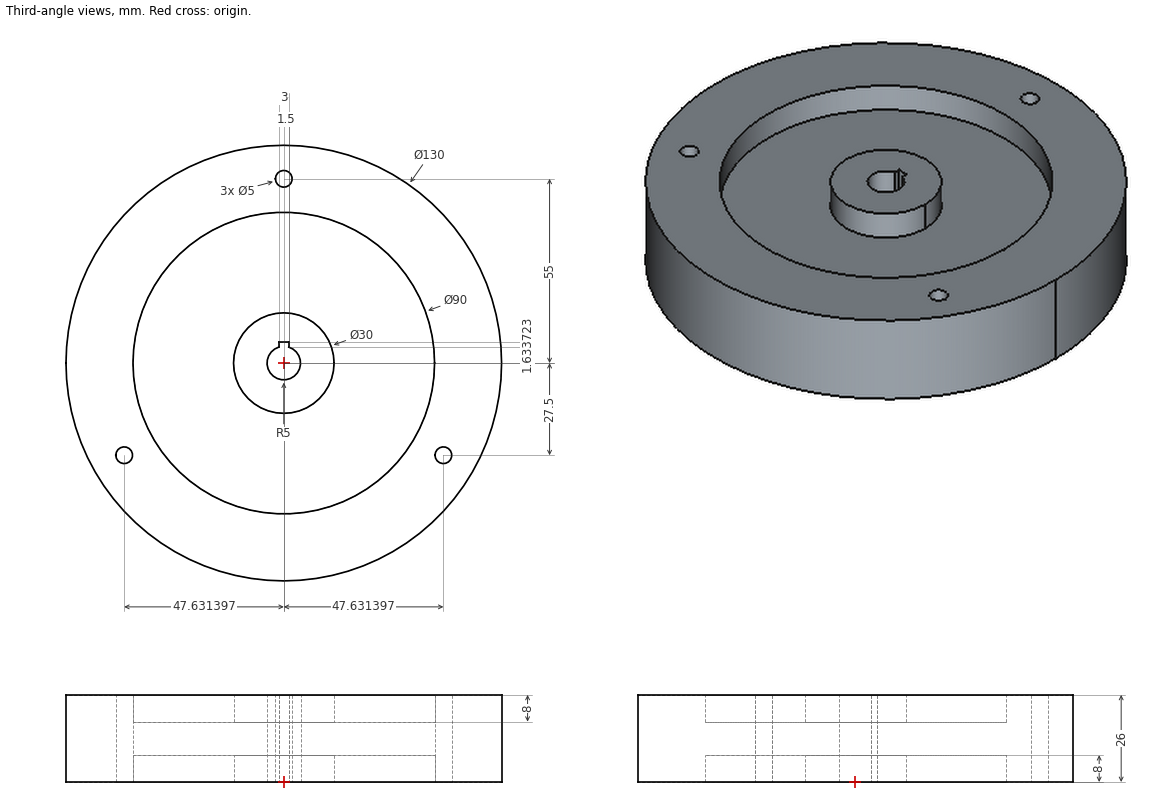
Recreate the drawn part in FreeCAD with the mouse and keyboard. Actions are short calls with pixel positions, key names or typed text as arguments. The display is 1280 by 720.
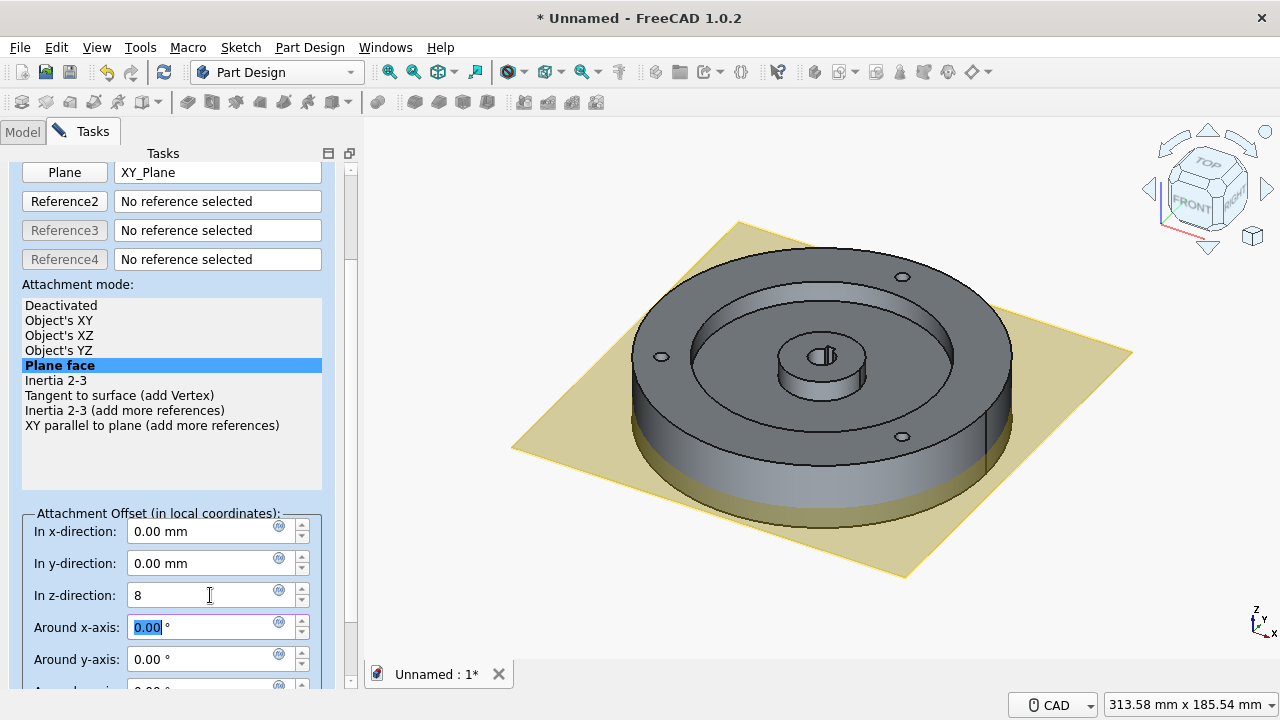
scroll(351, 426, up, 3)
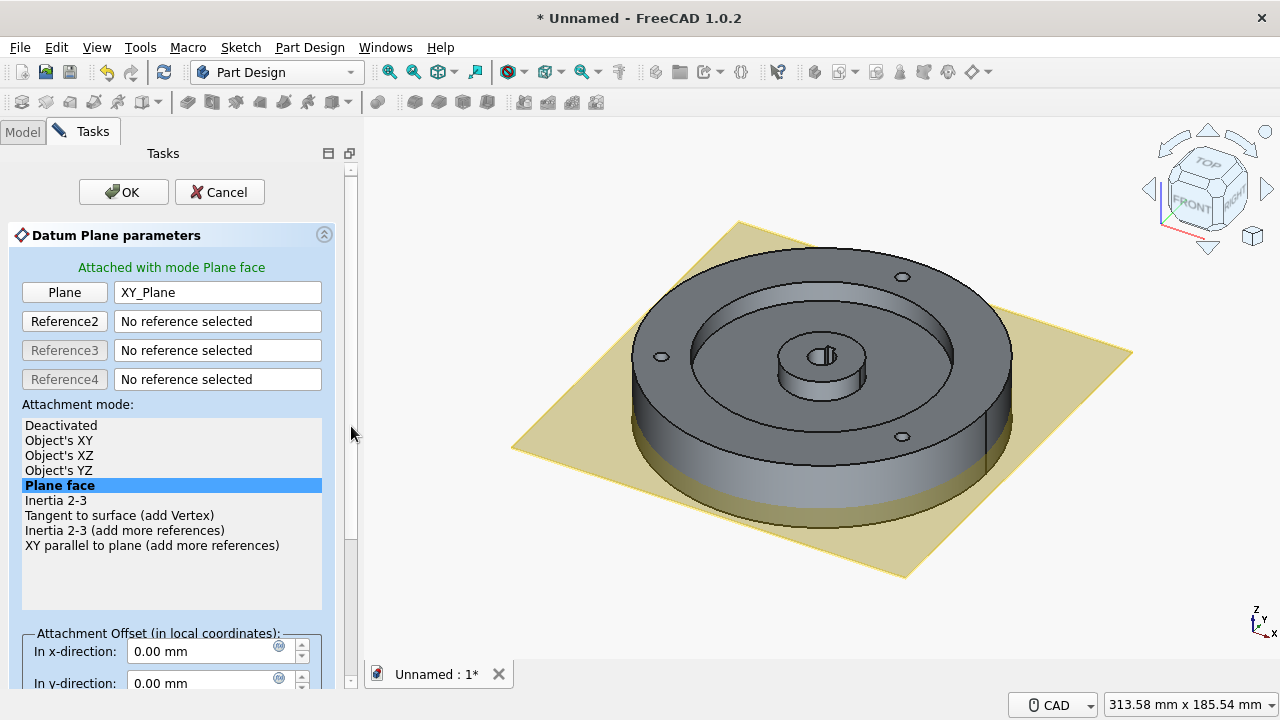
click(124, 192)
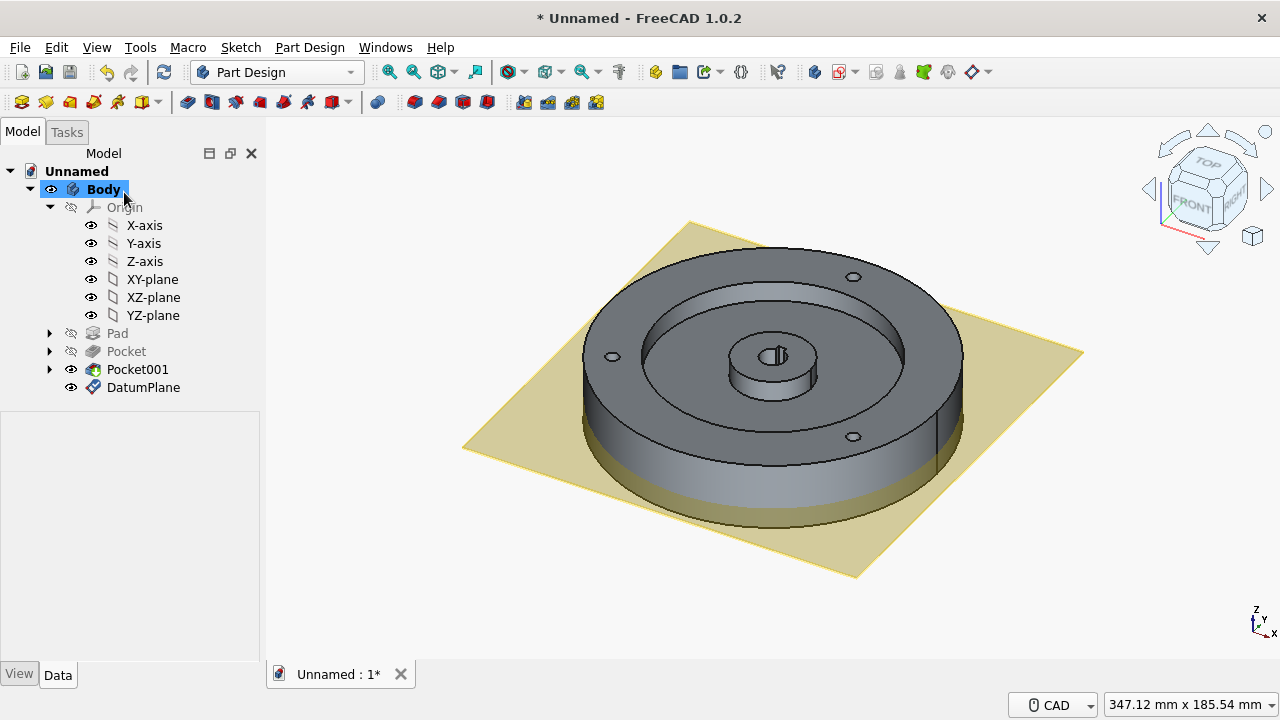
click(116, 387)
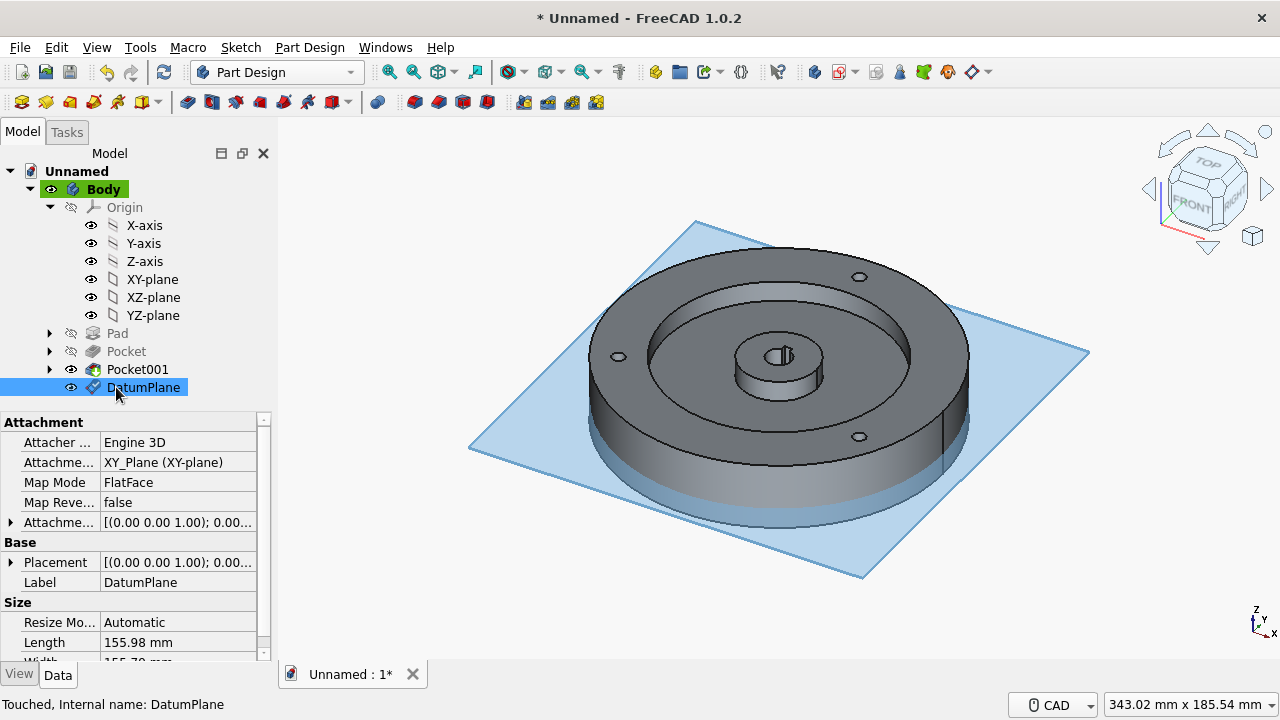
click(840, 72)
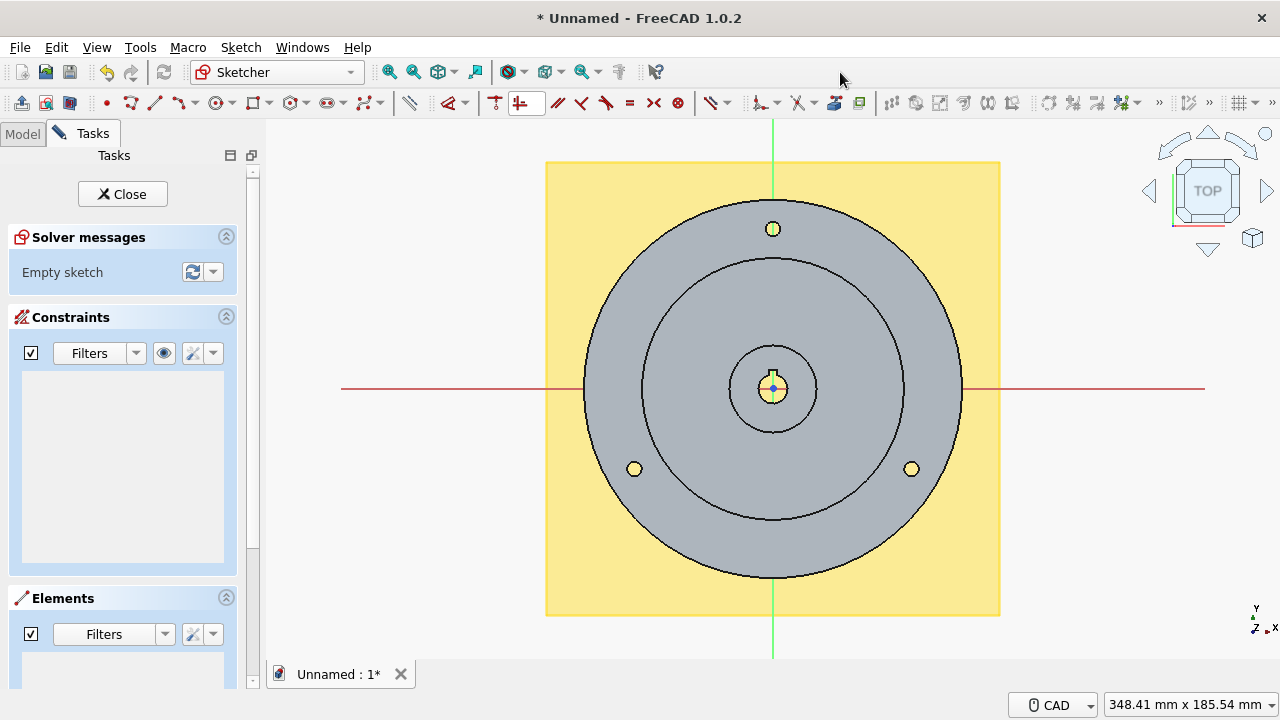
key(q)
key(s)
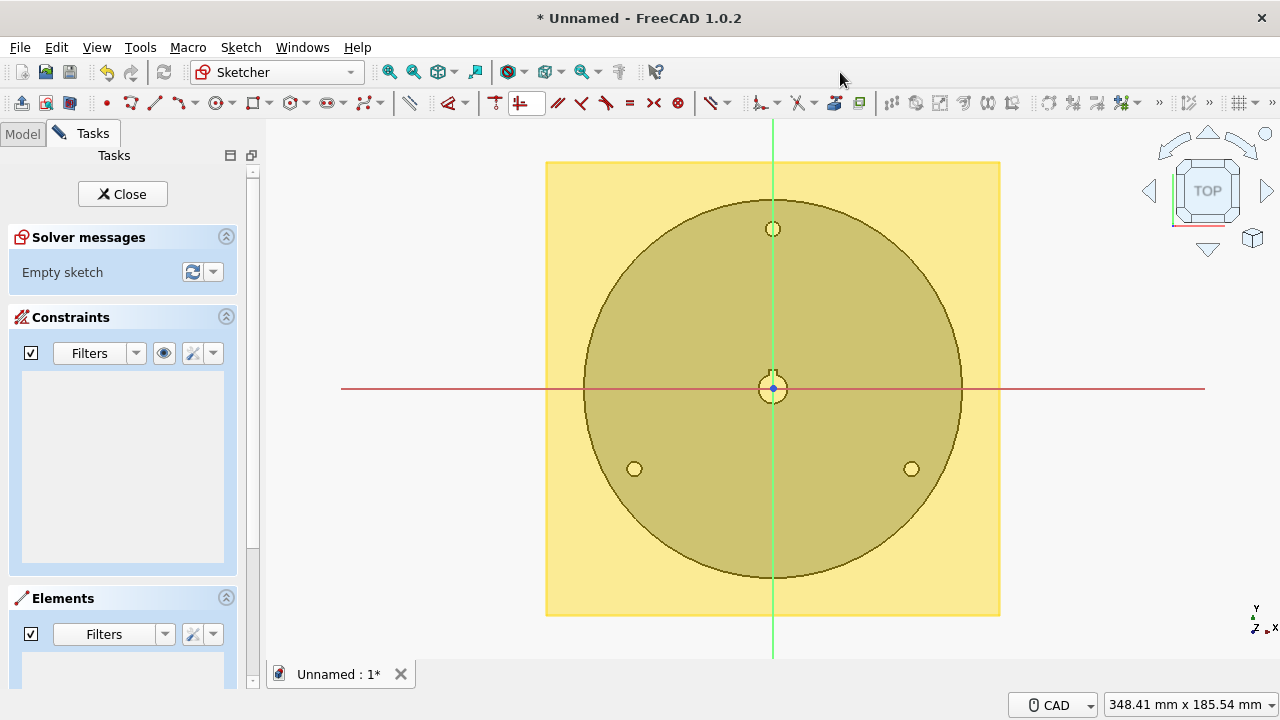
click(216, 104)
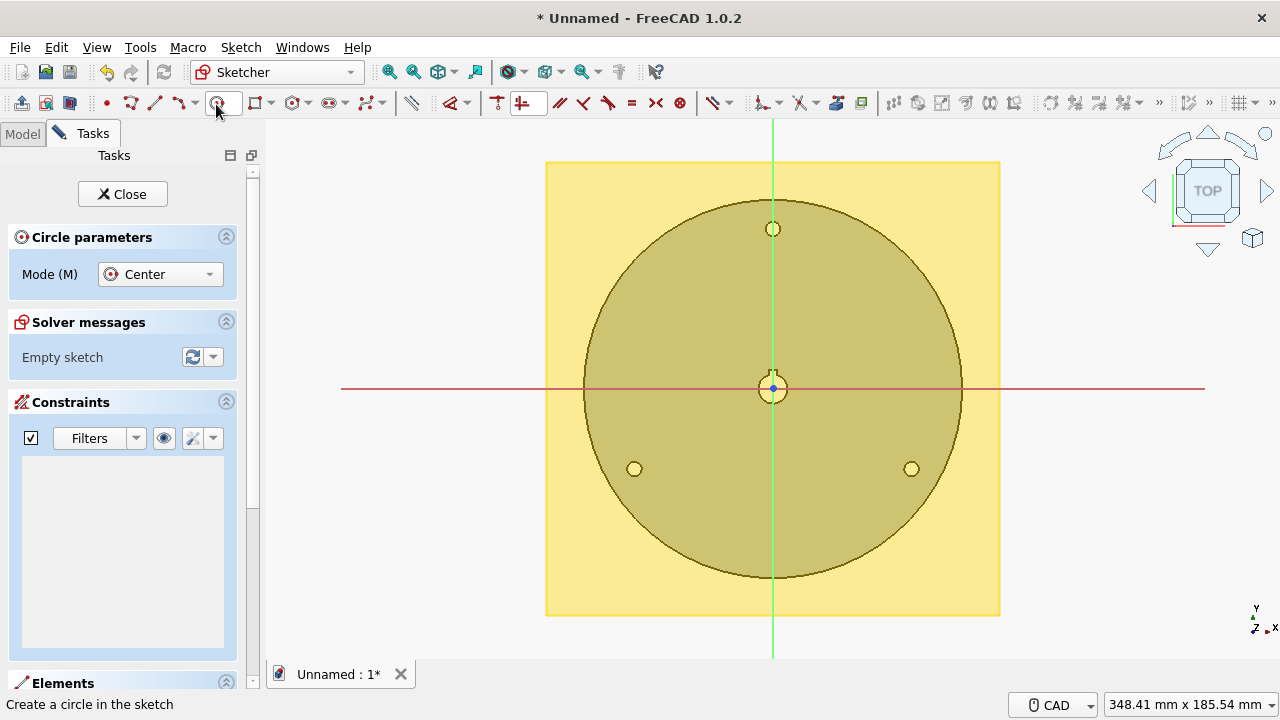
click(773, 389)
click(866, 296)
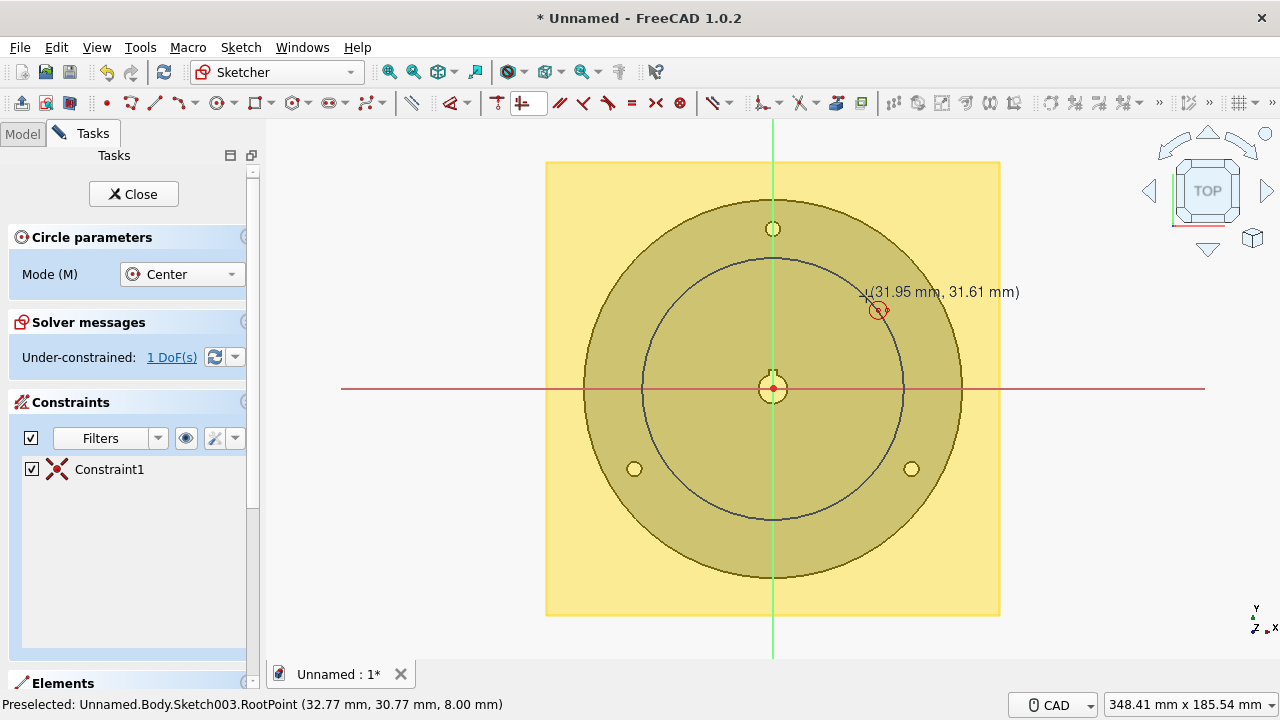
click(773, 389)
click(804, 358)
key(Escape)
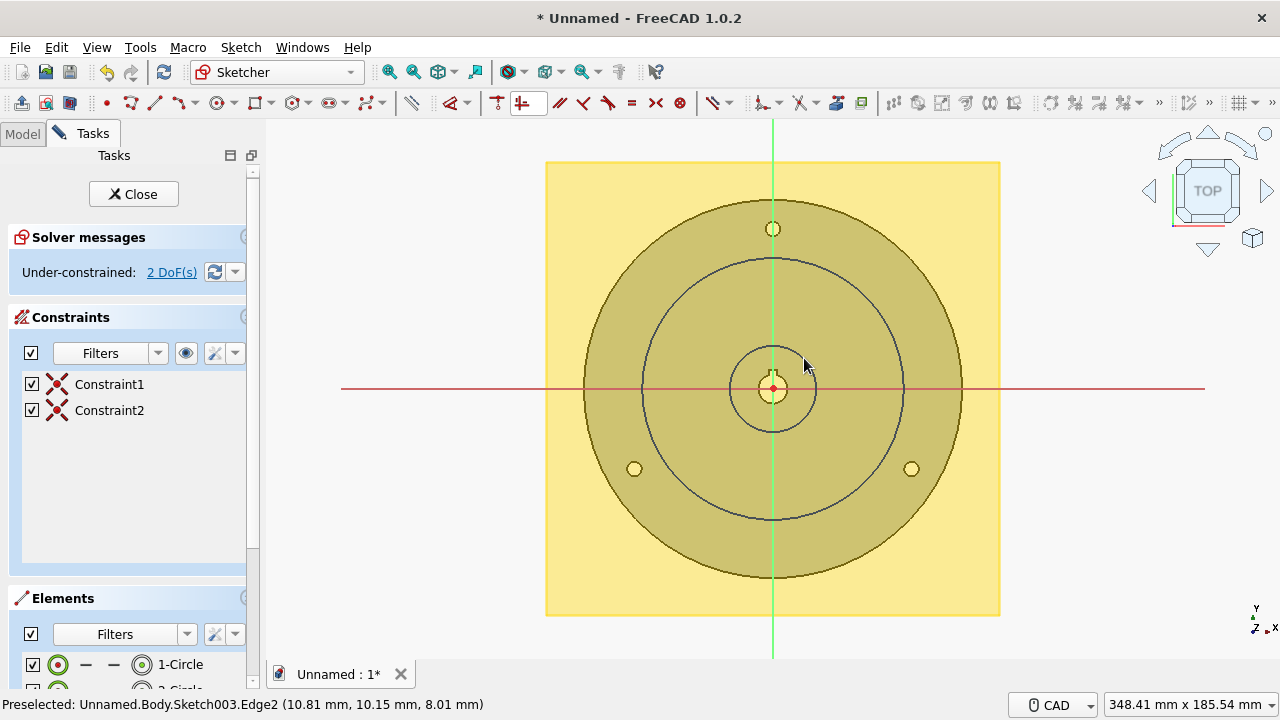
key(d)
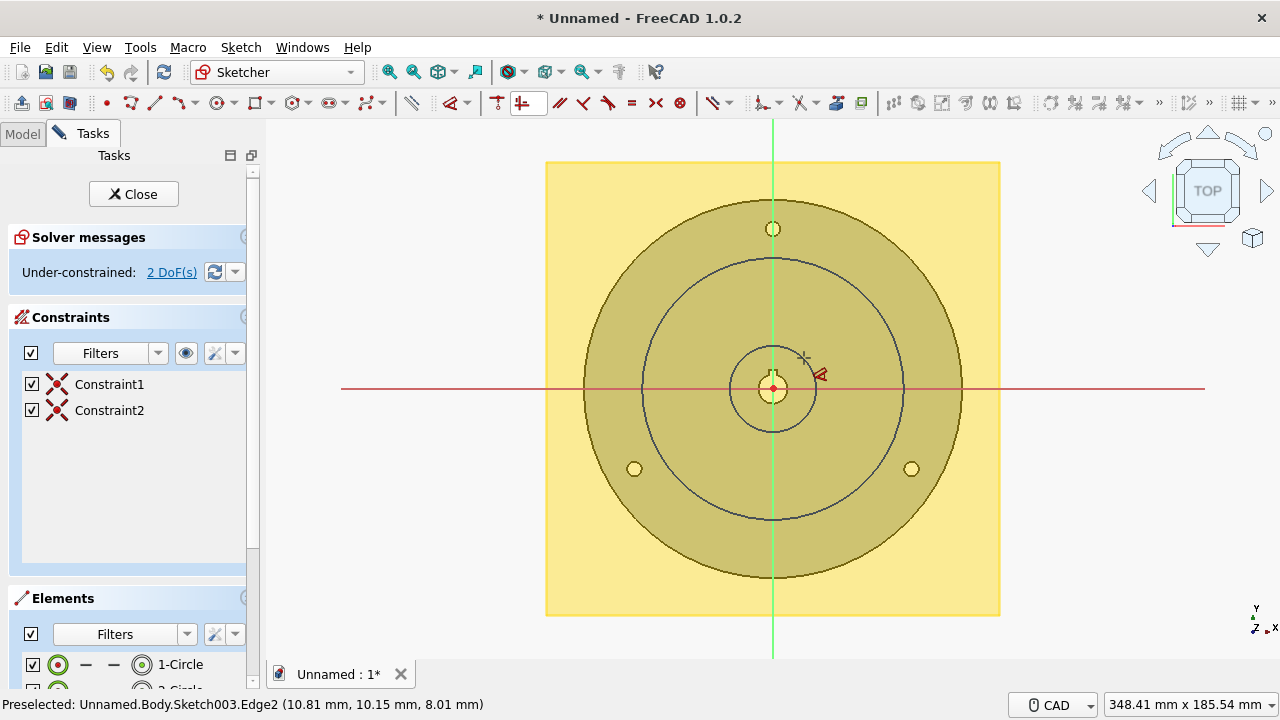
click(865, 296)
click(888, 273)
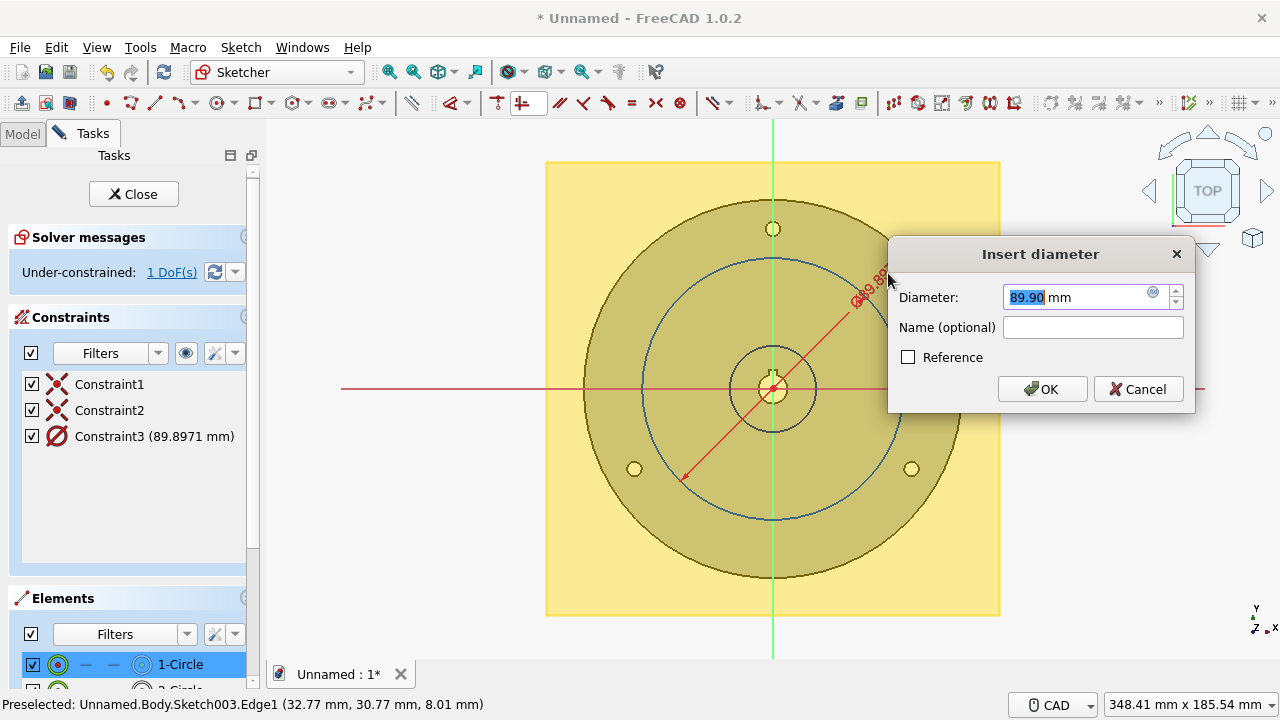
text(90)
key(Return)